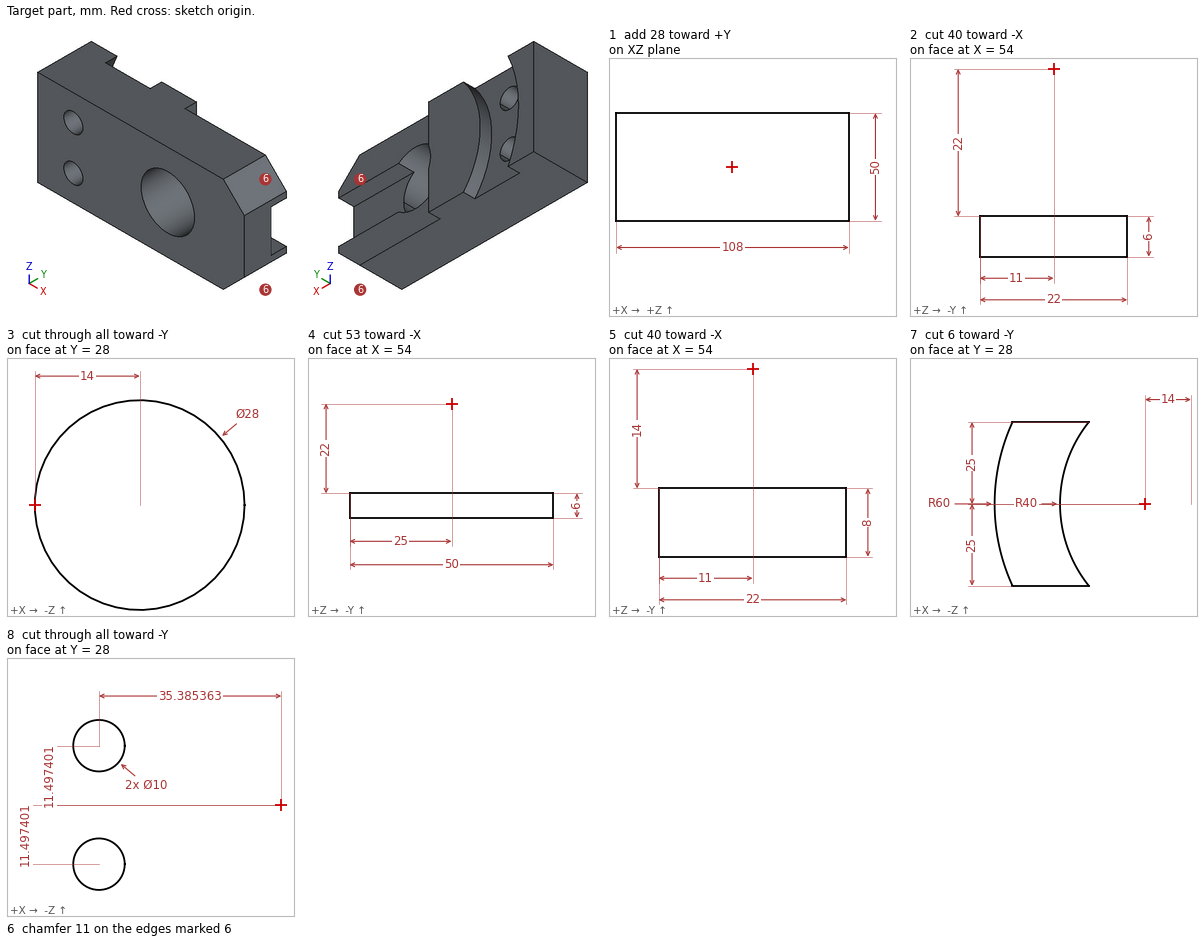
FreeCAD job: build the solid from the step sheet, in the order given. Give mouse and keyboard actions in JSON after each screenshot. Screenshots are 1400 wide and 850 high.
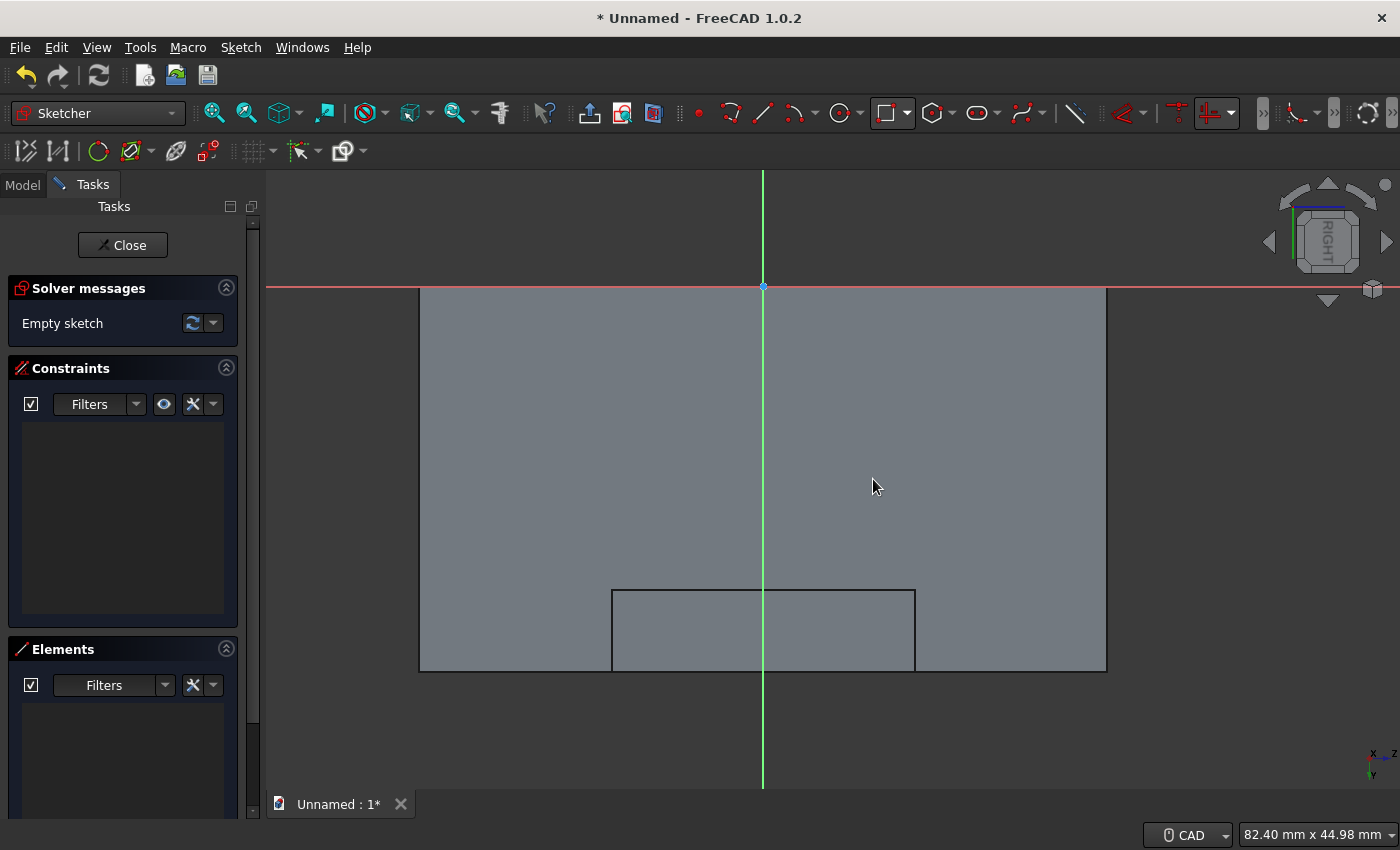
{"action": "key", "text": "g r"}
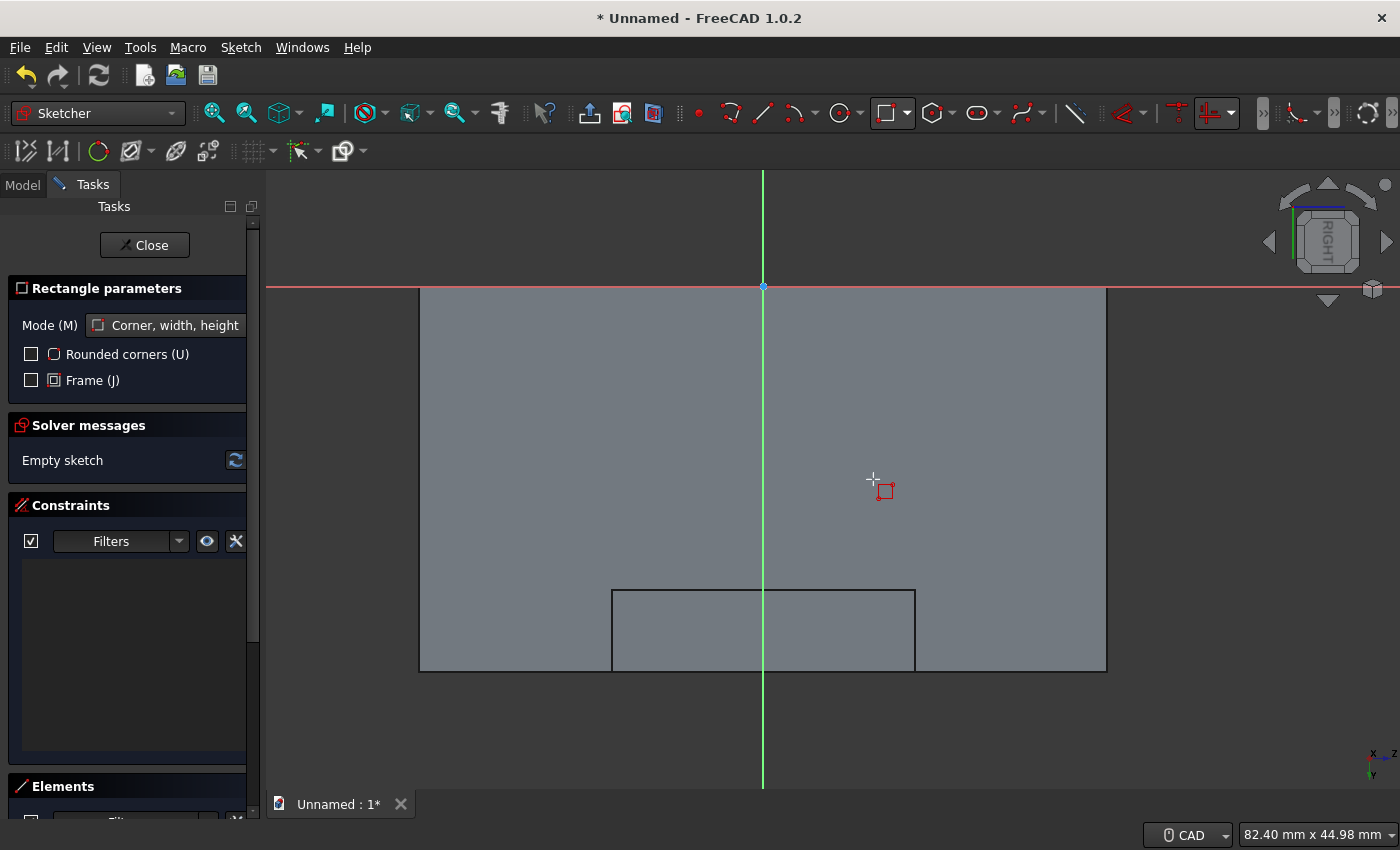
{"action": "left_click", "coordinate": [419, 590]}
{"action": "mouse_move", "coordinate": [1107, 672]}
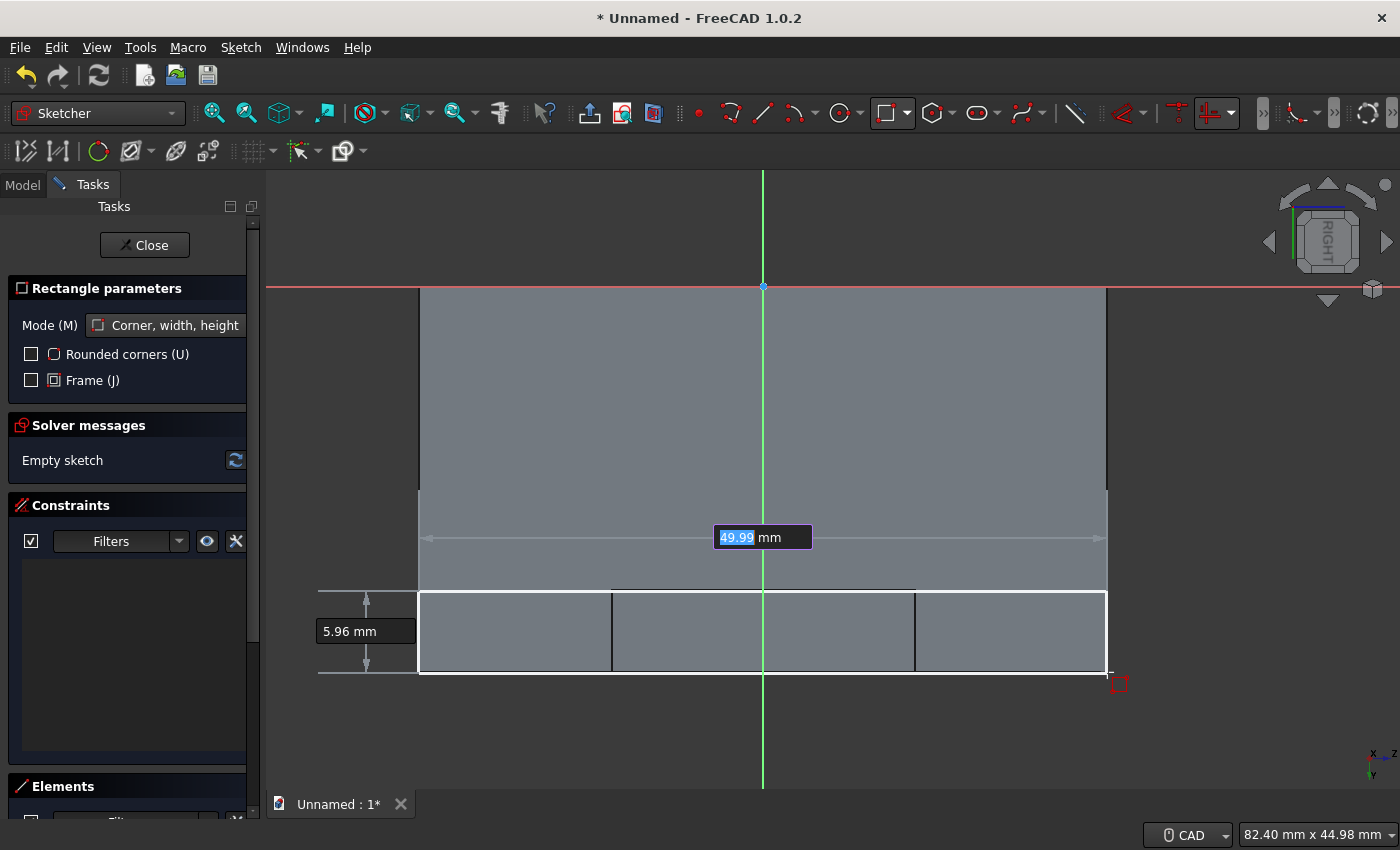
{"action": "type", "text": "50"}
{"action": "key", "text": "Tab"}
{"action": "type", "text": "6"}
{"action": "key", "text": "Return"}
{"action": "key", "text": "Escape"}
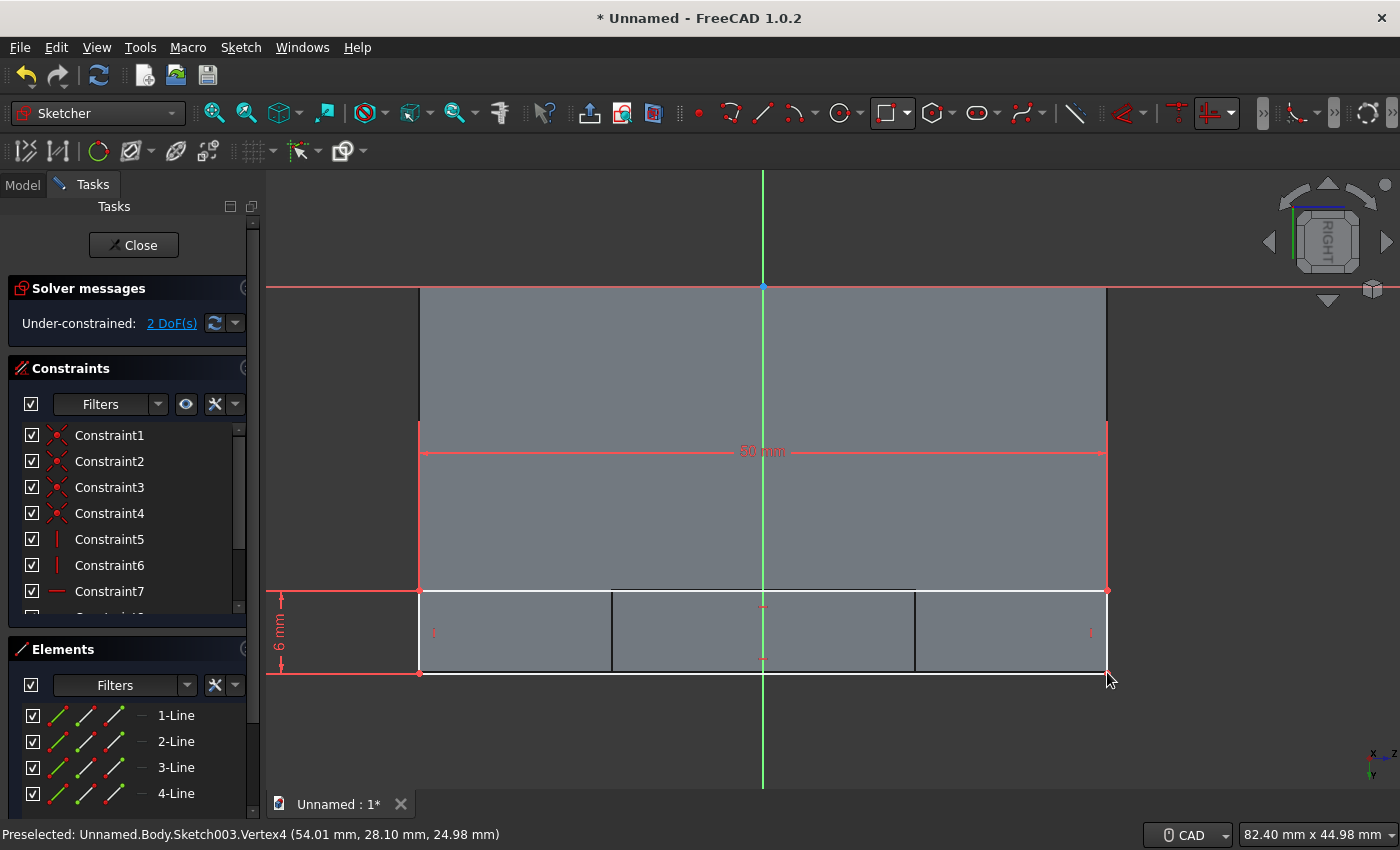
{"action": "left_click", "coordinate": [1122, 114]}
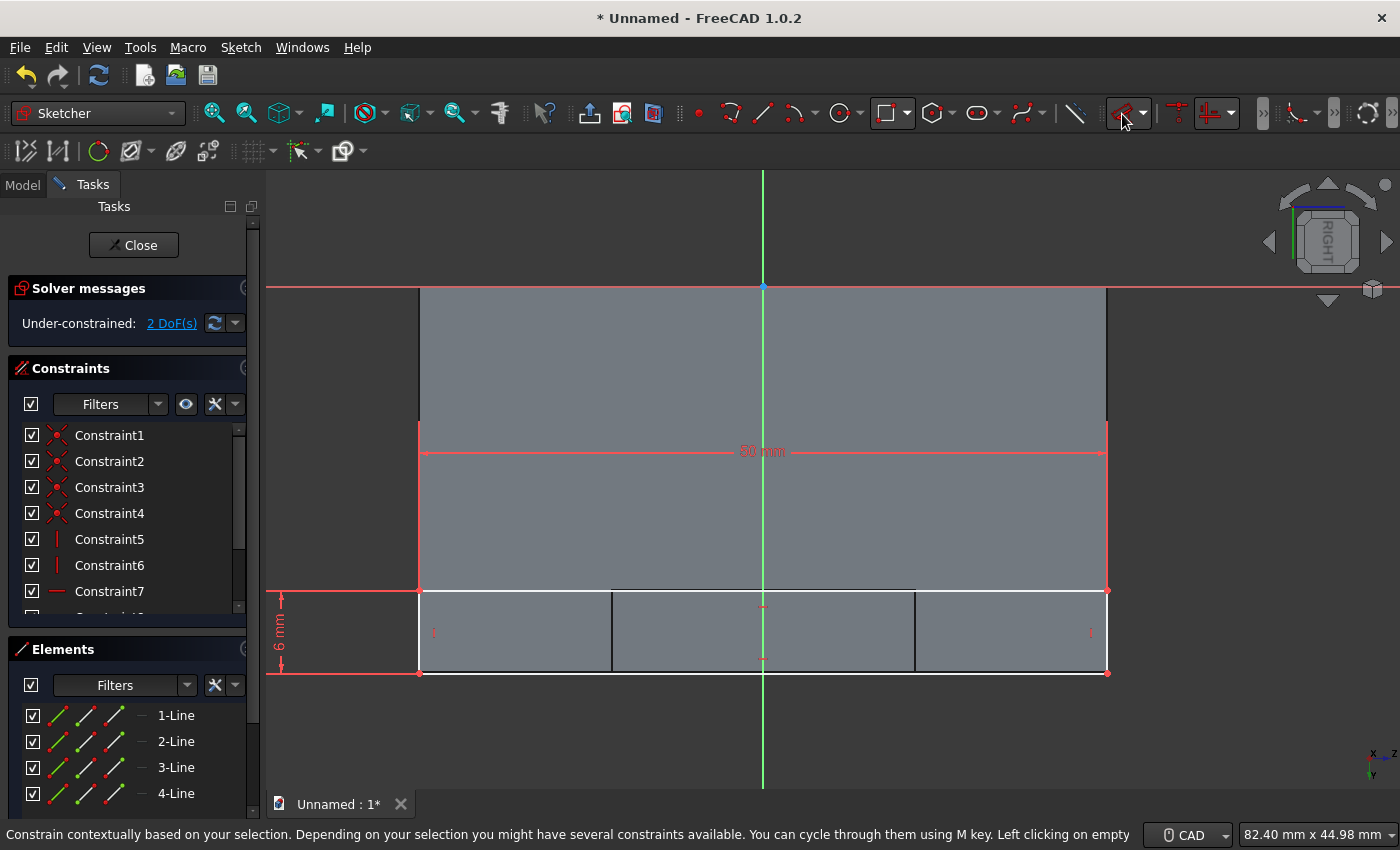
{"action": "left_click", "coordinate": [419, 591]}
{"action": "left_click", "coordinate": [591, 253]}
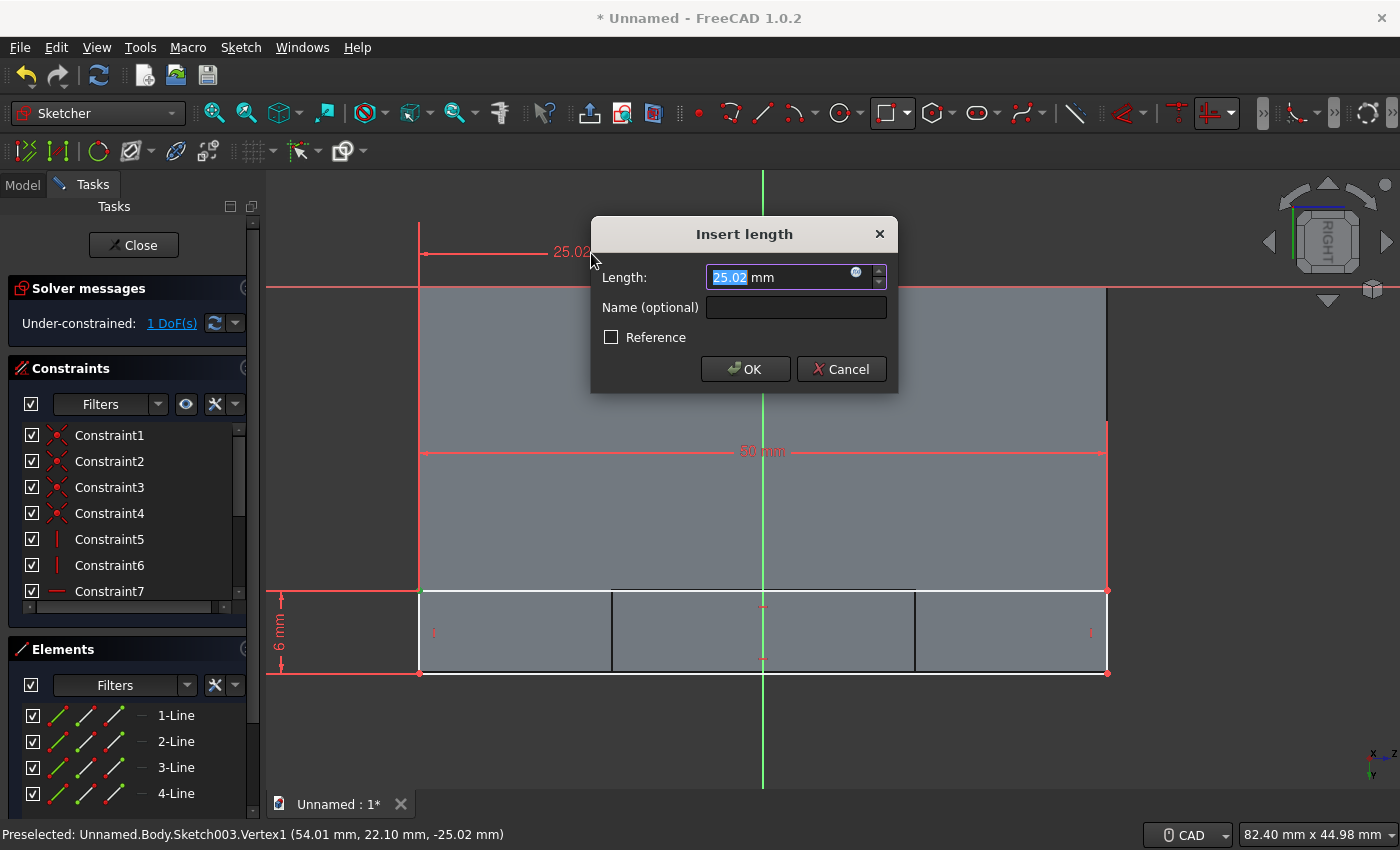
{"action": "type", "text": "25"}
{"action": "key", "text": "Return"}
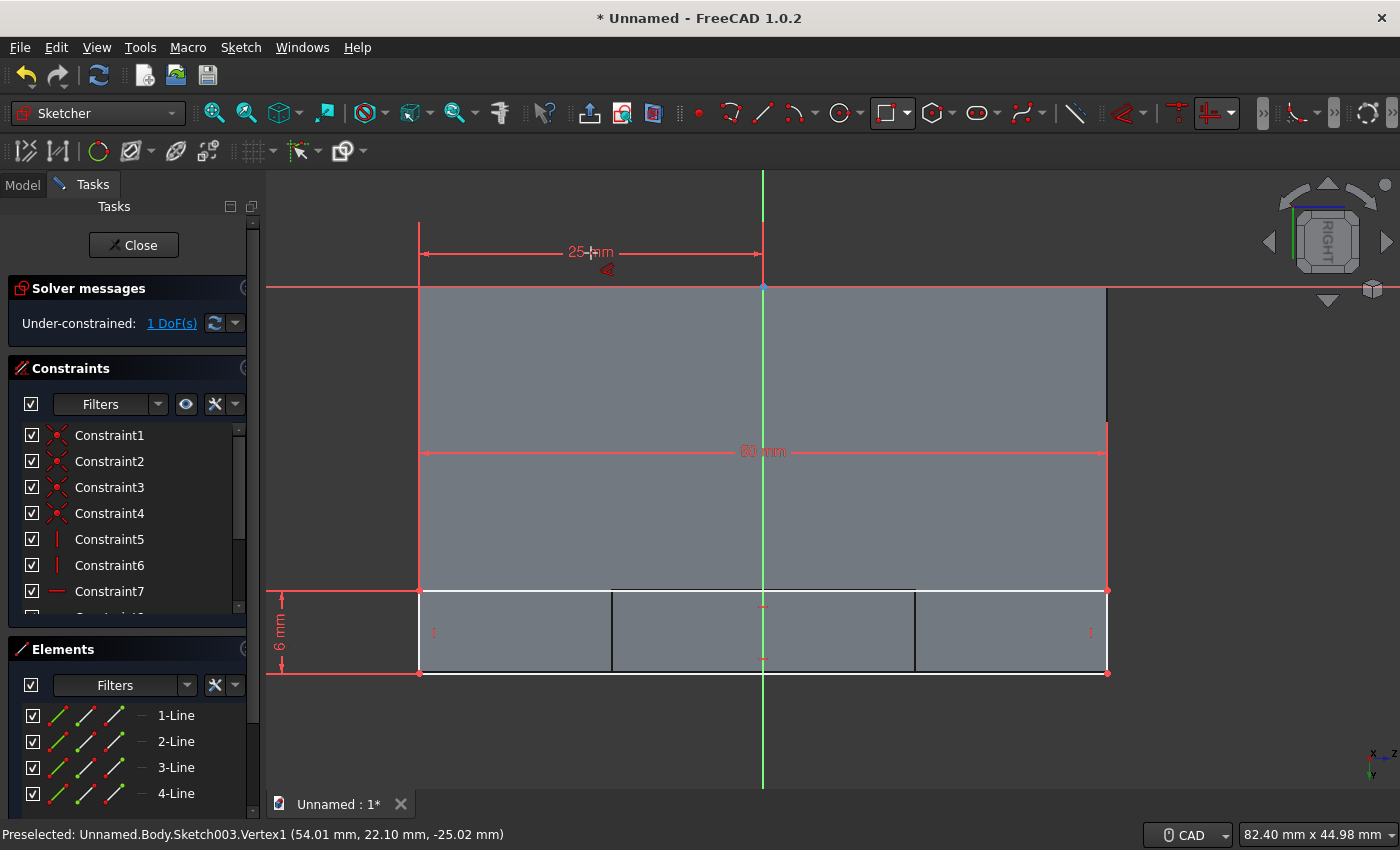
{"action": "left_click", "coordinate": [419, 591]}
{"action": "left_click", "coordinate": [385, 439]}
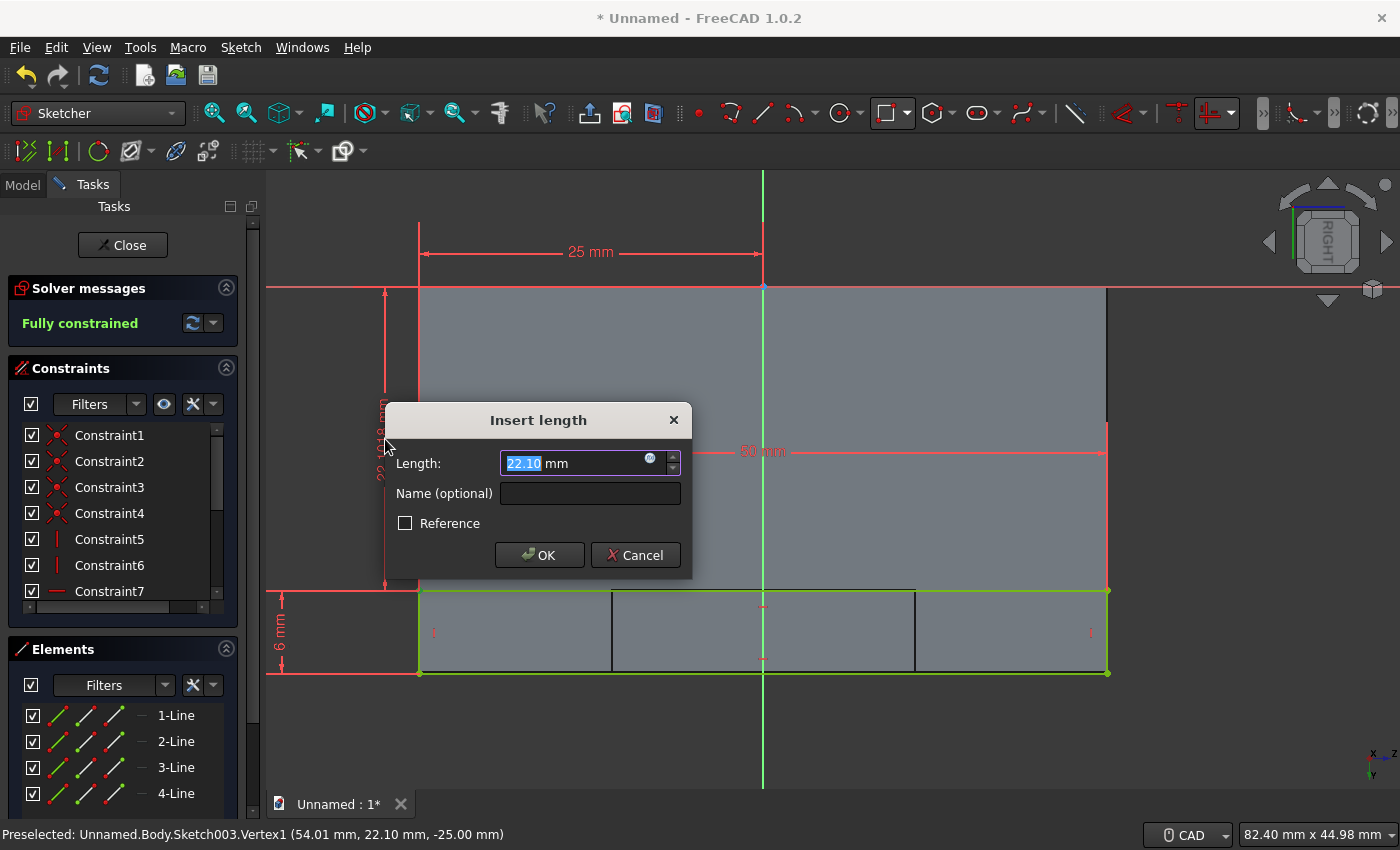
{"action": "type", "text": "22"}
{"action": "key", "text": "Return"}
{"action": "key", "text": "Escape"}